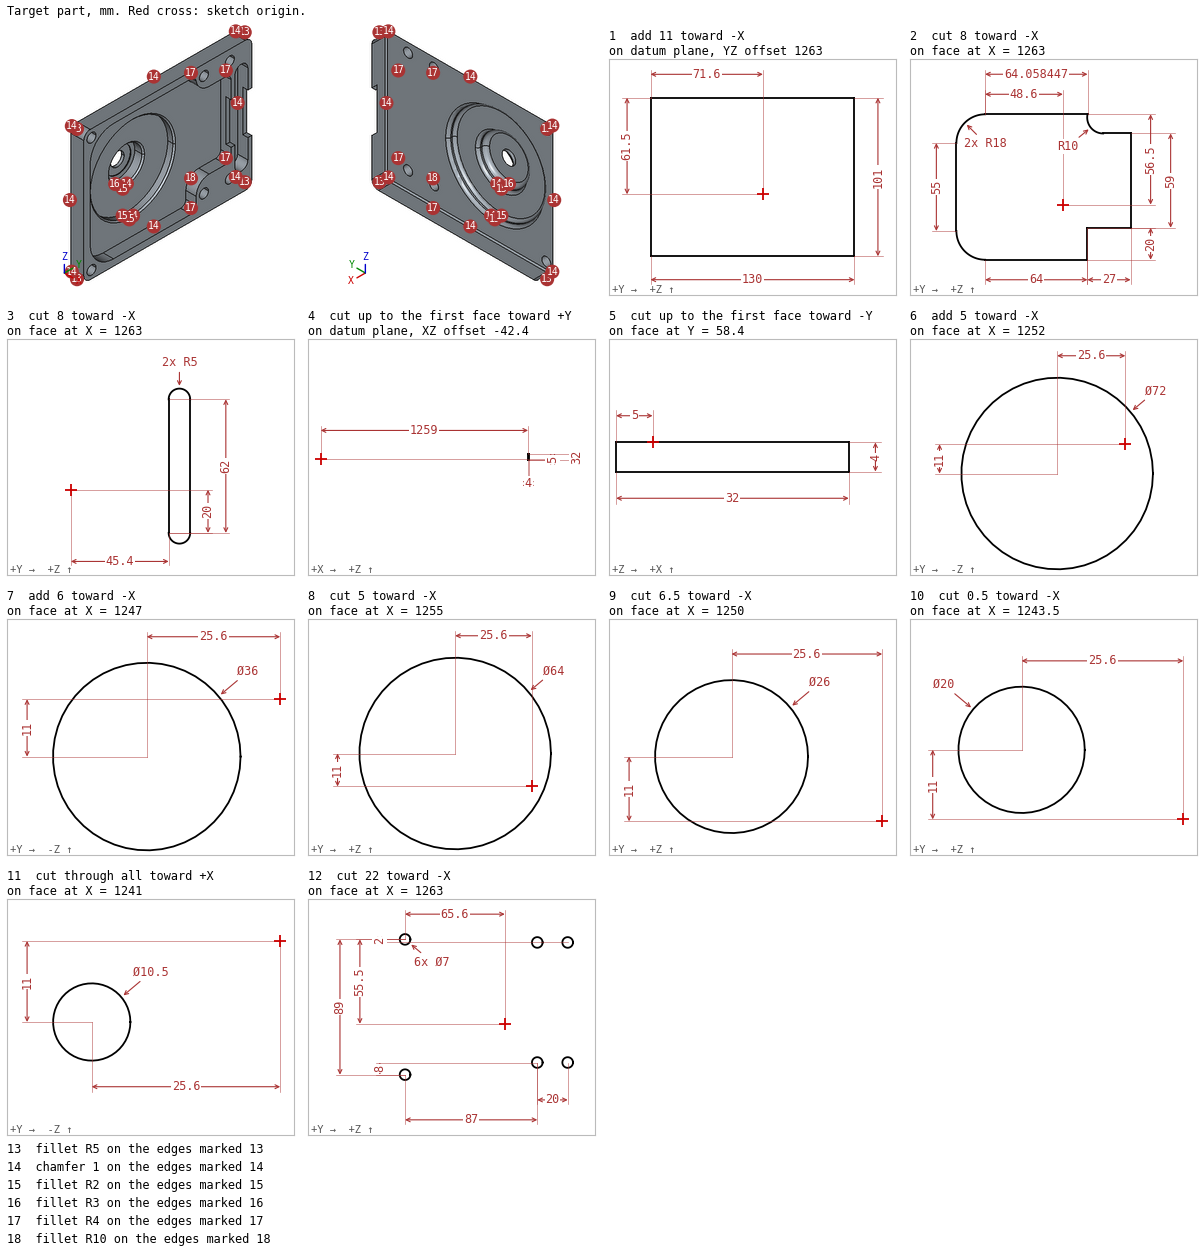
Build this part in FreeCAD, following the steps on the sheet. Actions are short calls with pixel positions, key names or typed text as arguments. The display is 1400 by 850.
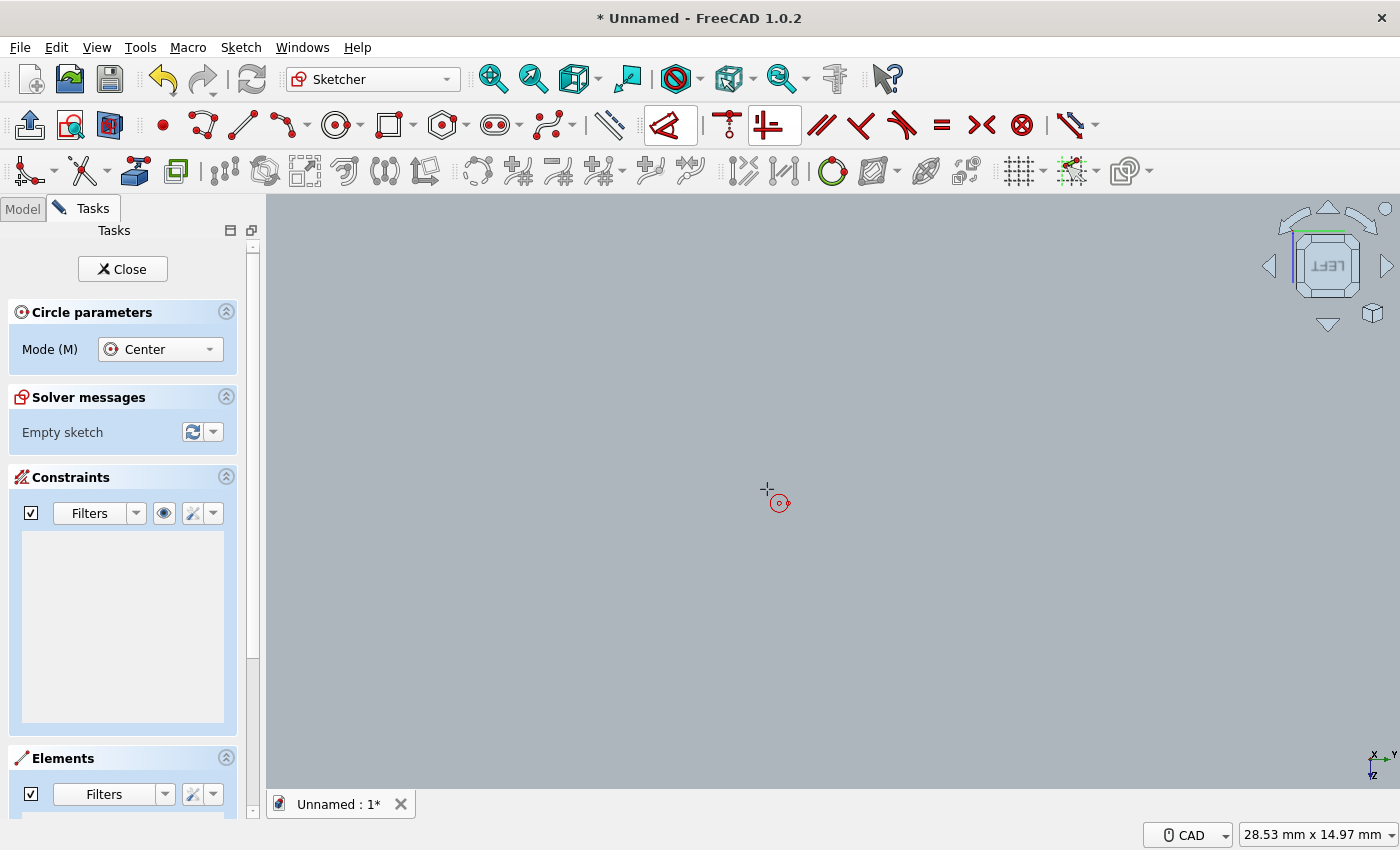
click(761, 485)
move(909, 338)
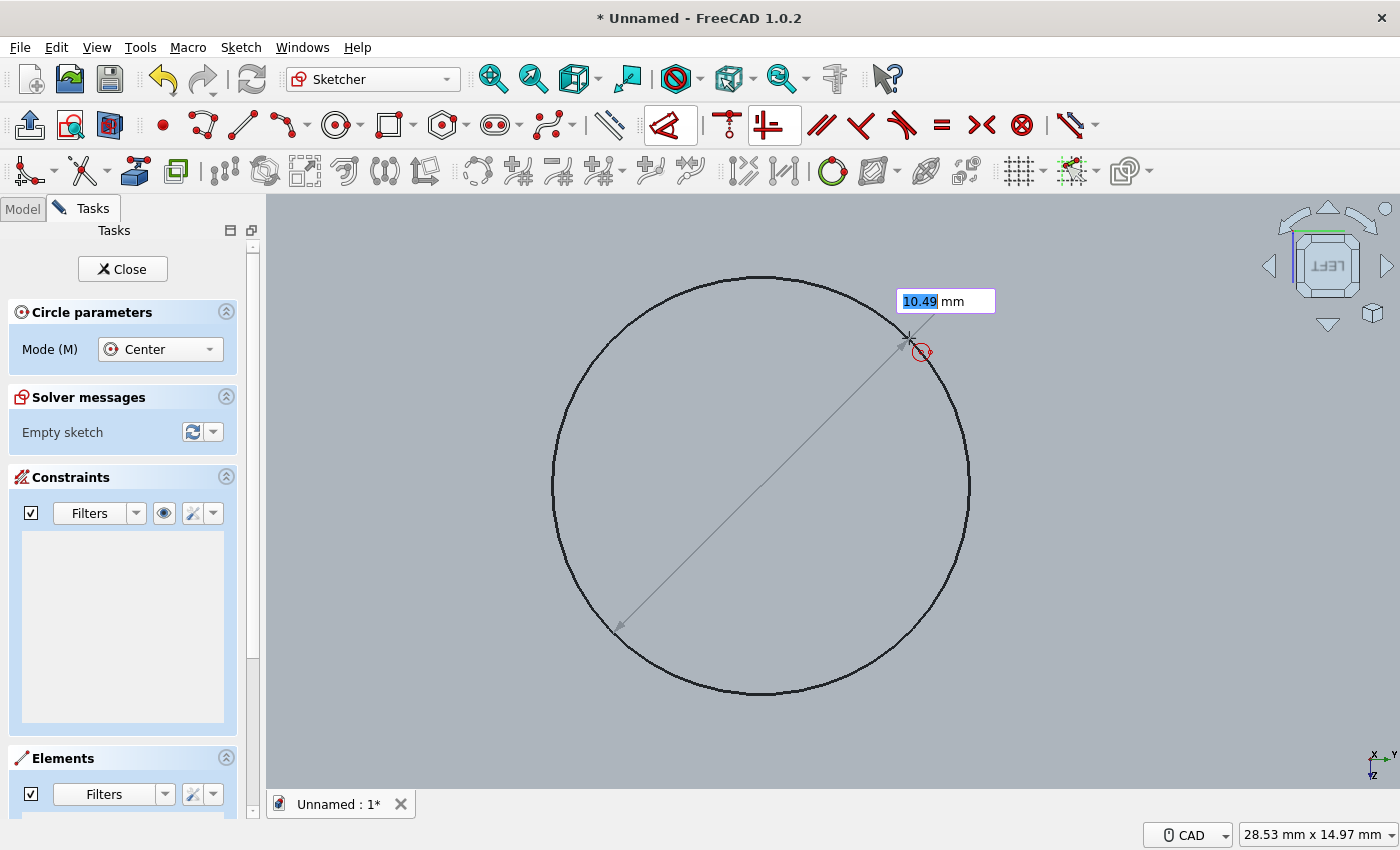
text(10.5)
key(Return)
key(Escape)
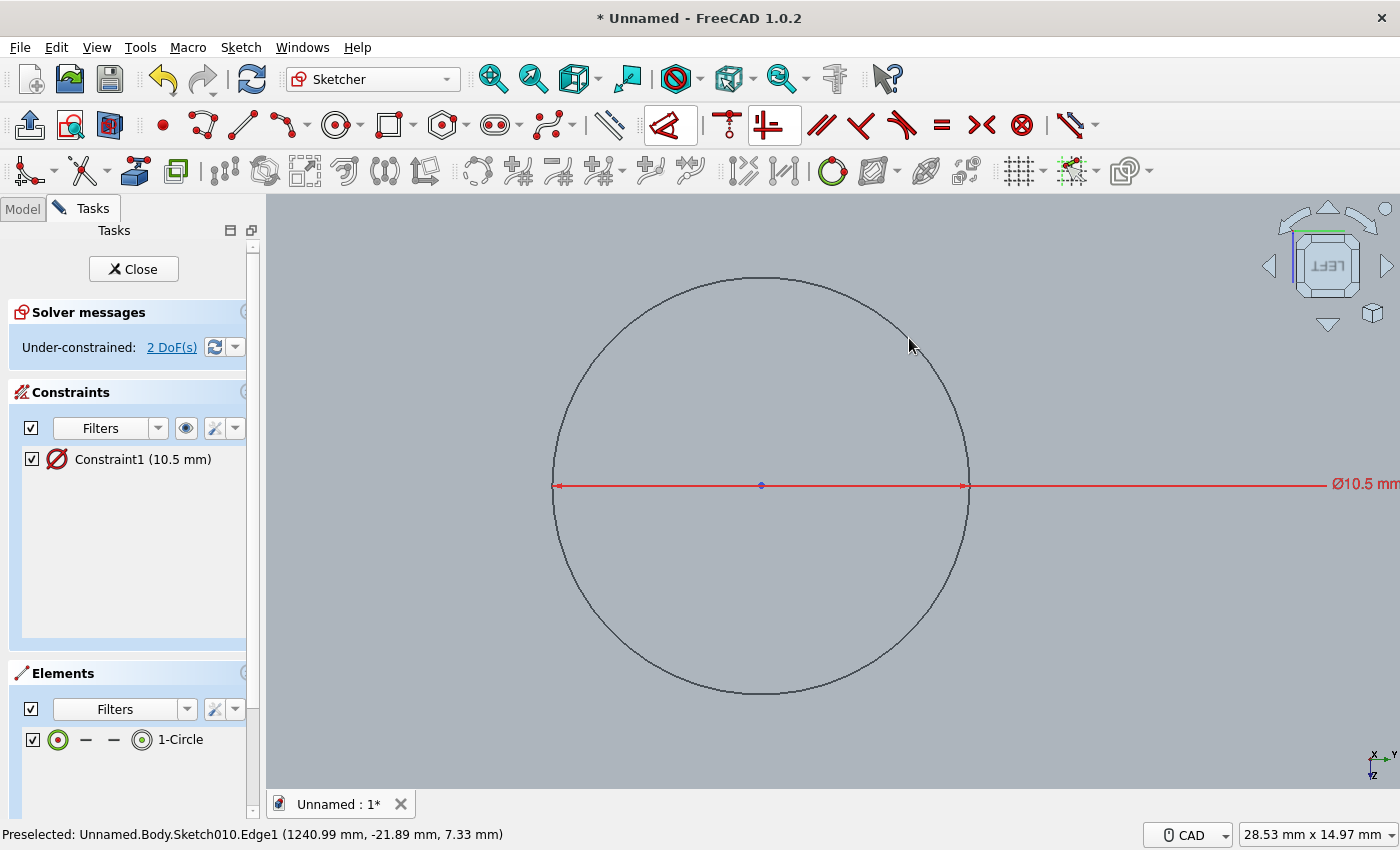
click(761, 486)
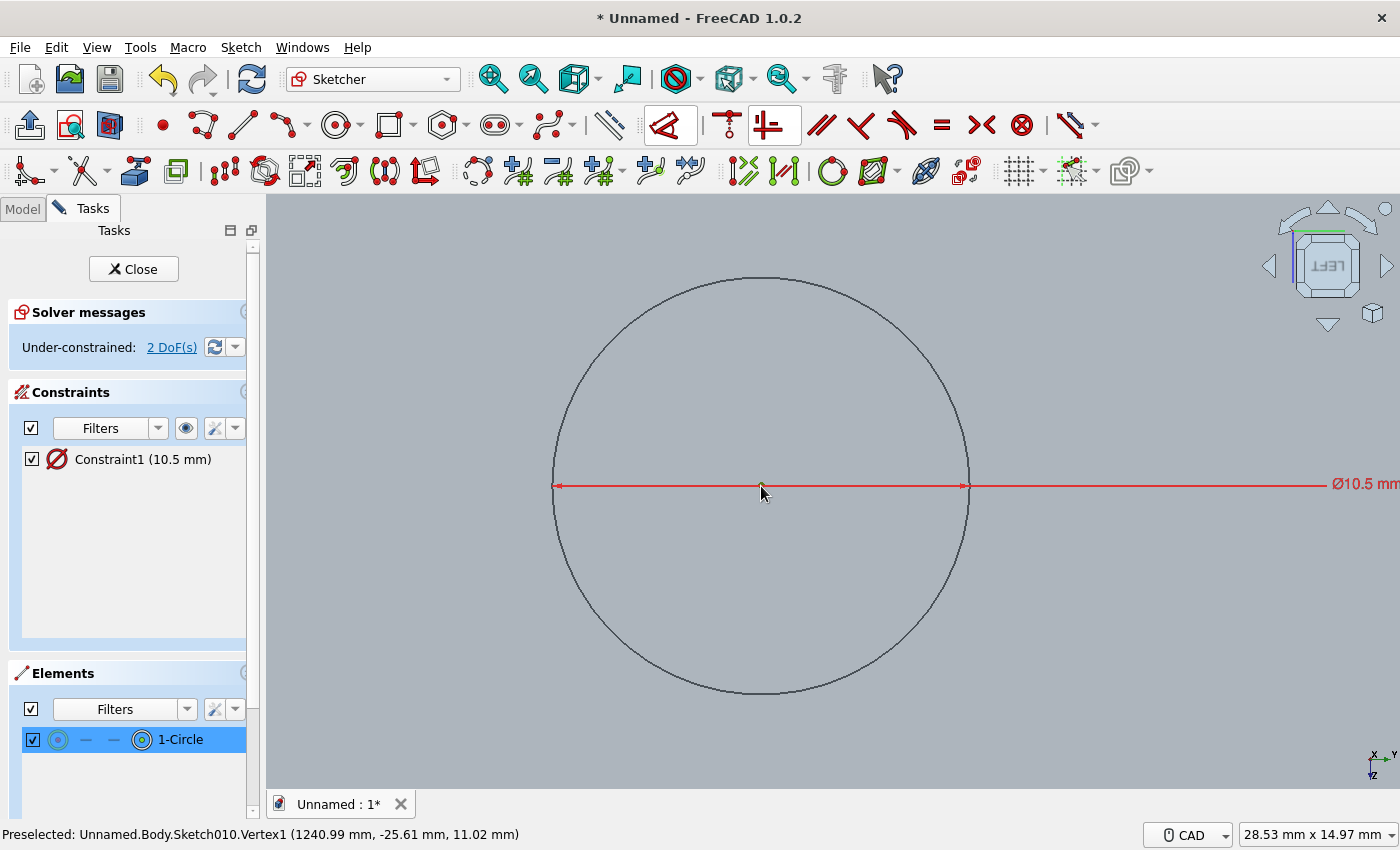
key(i)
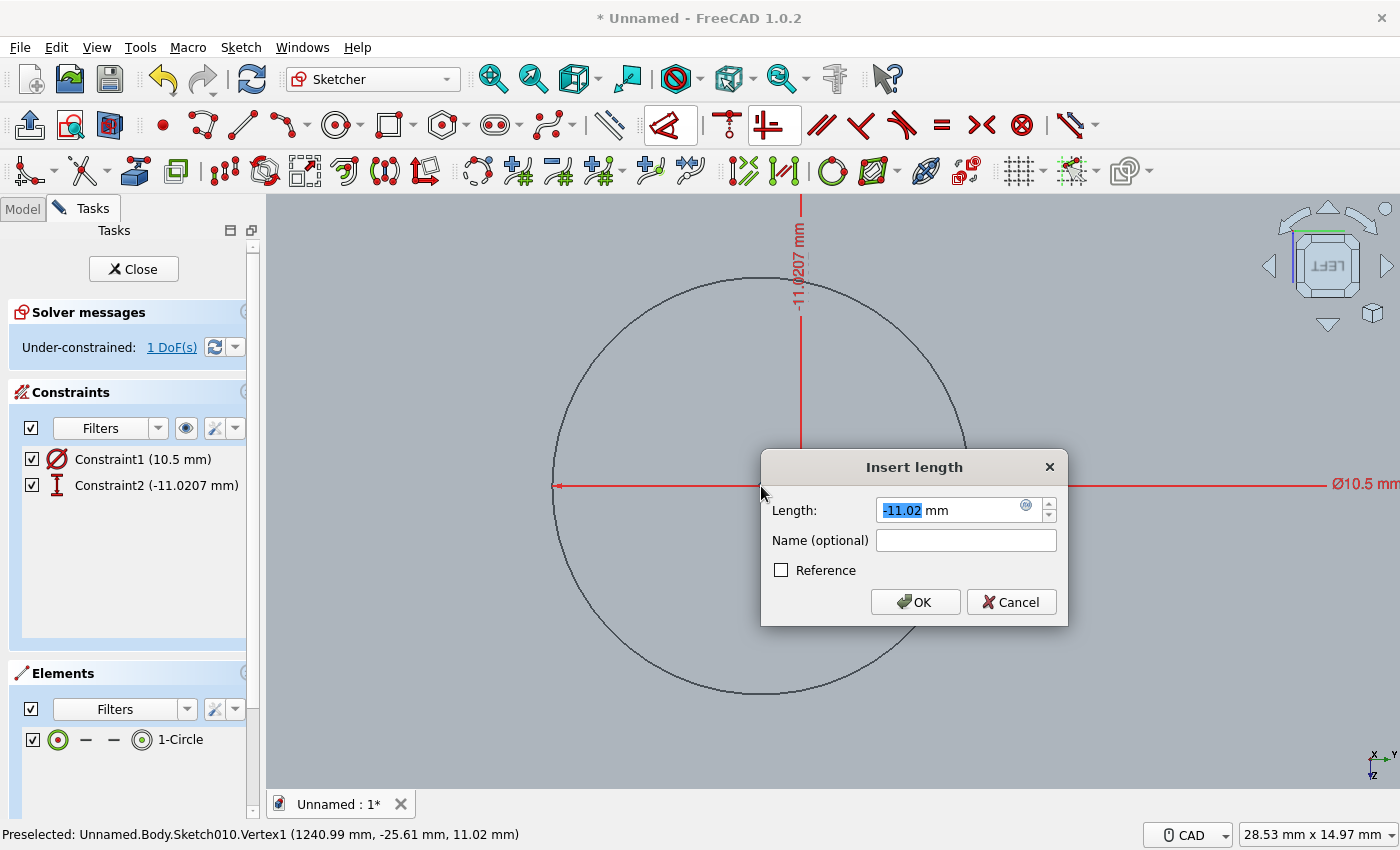
text(-11)
key(Return)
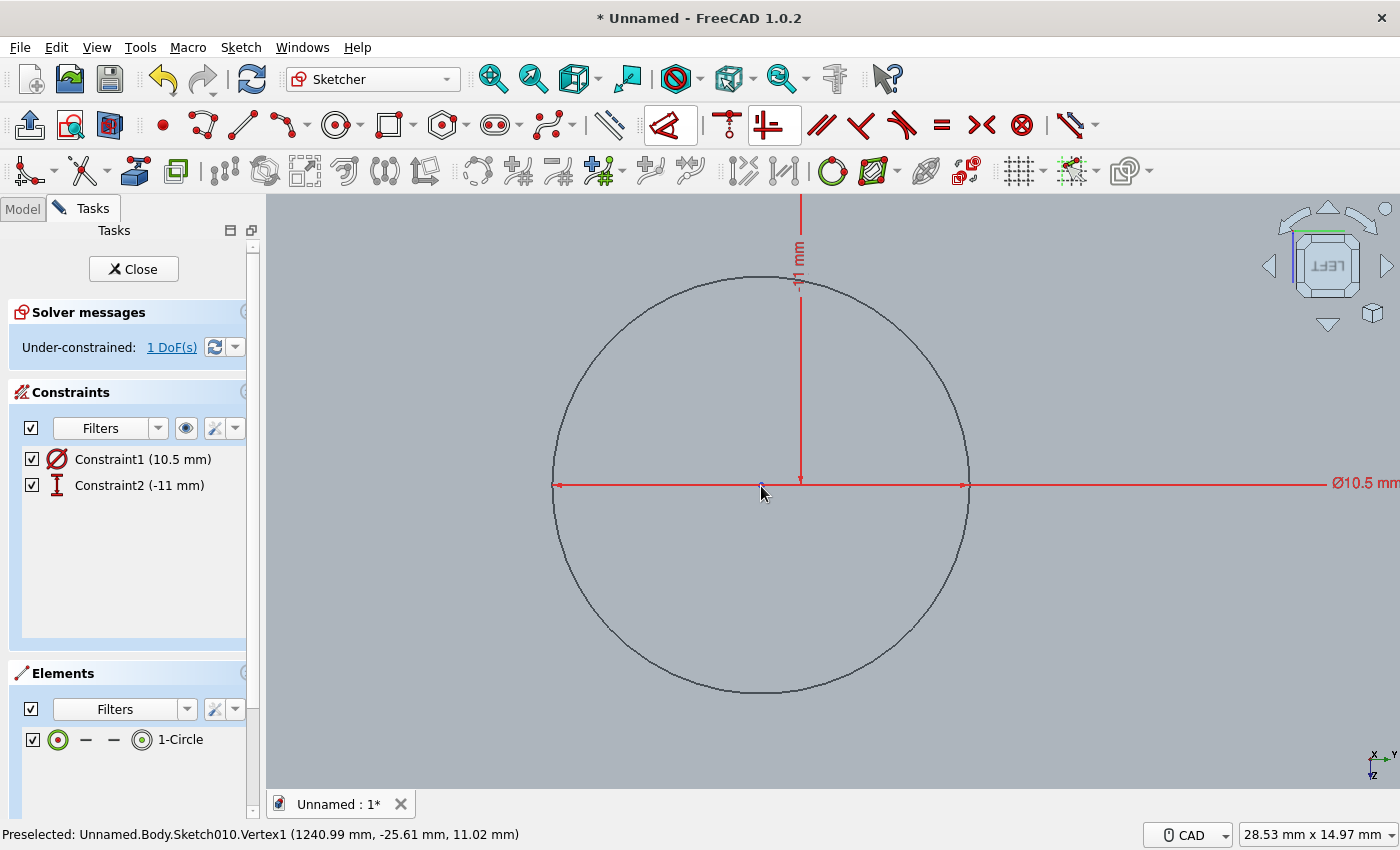
click(761, 485)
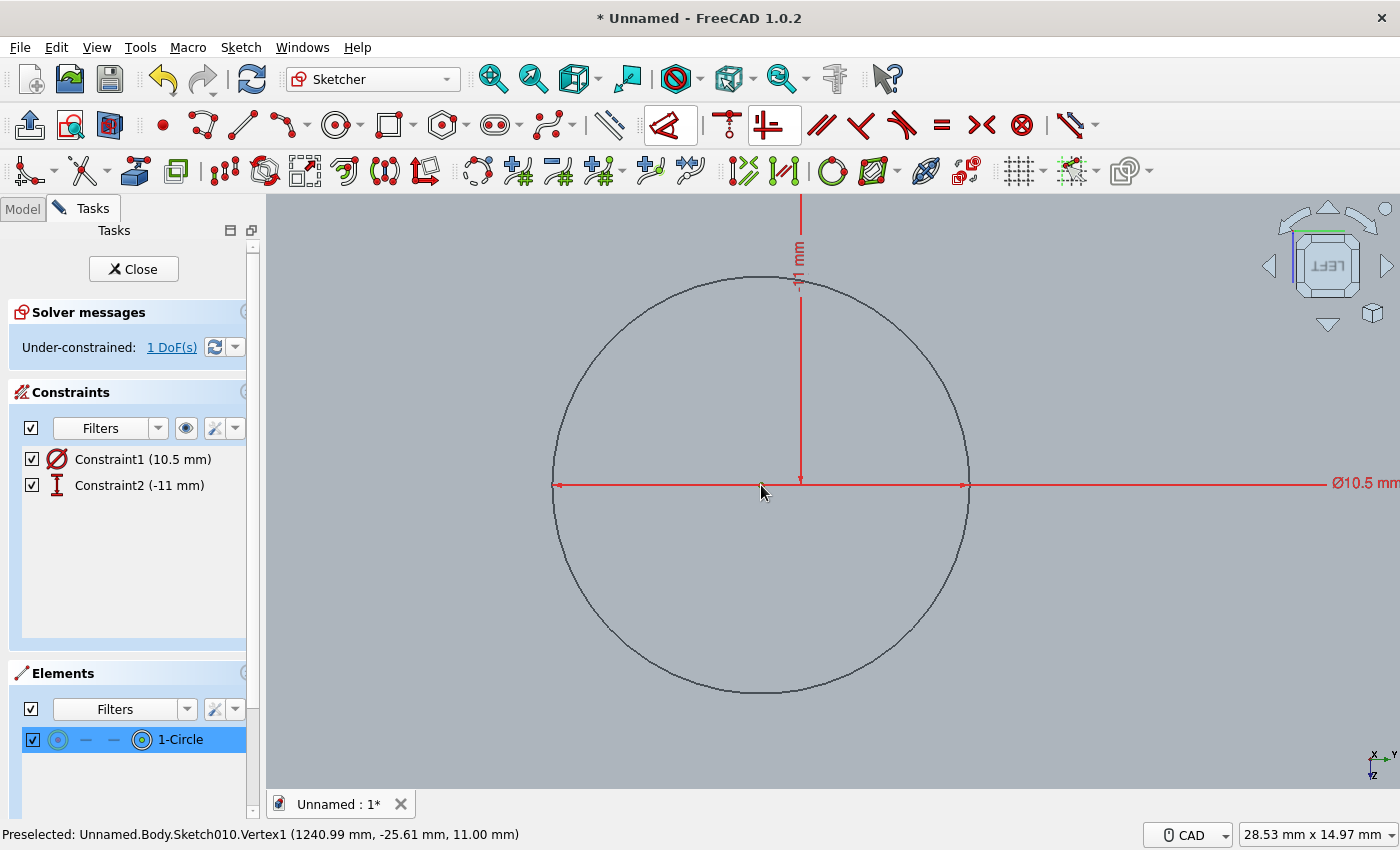
key(l)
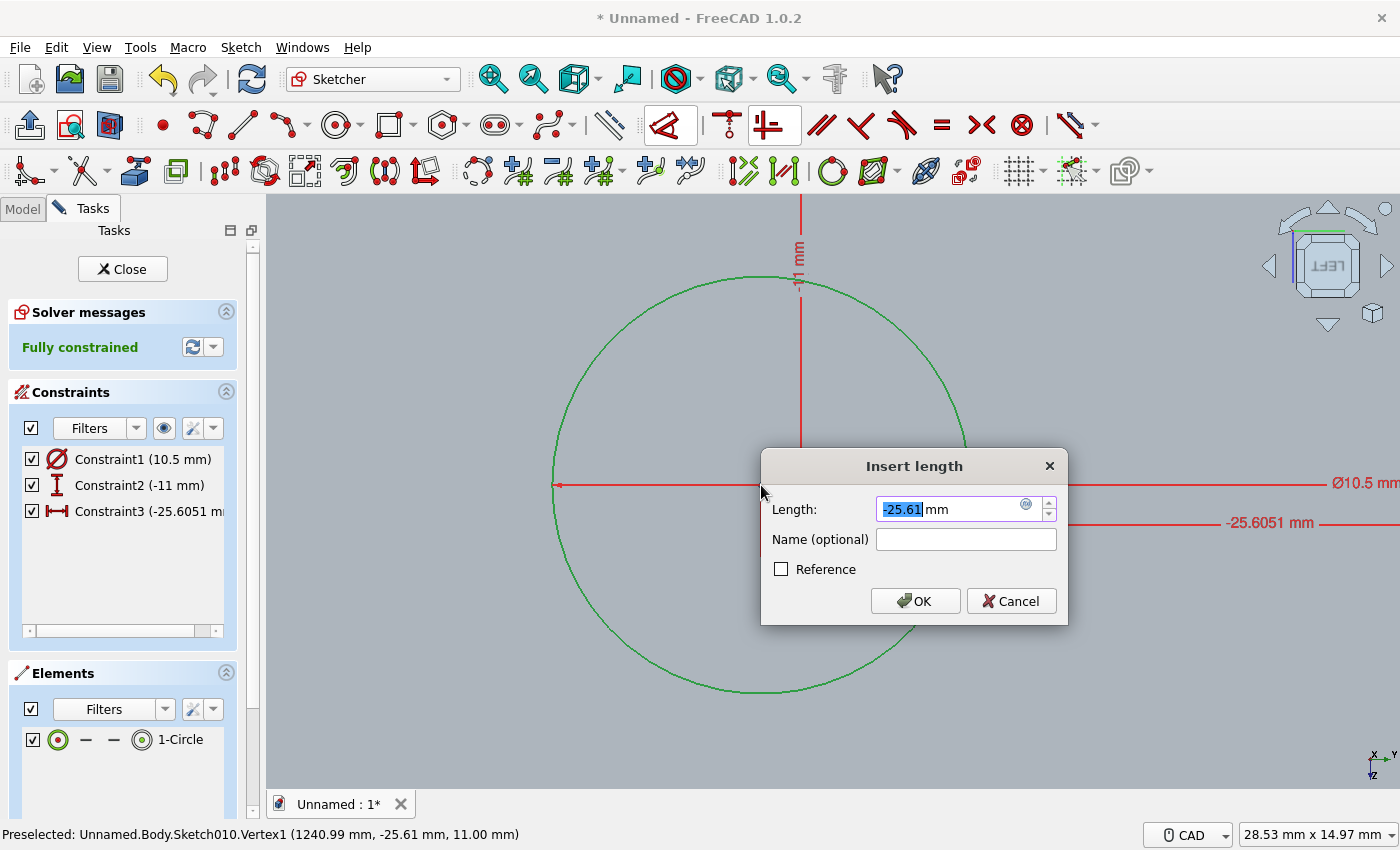
text(-25.6)
key(Return)